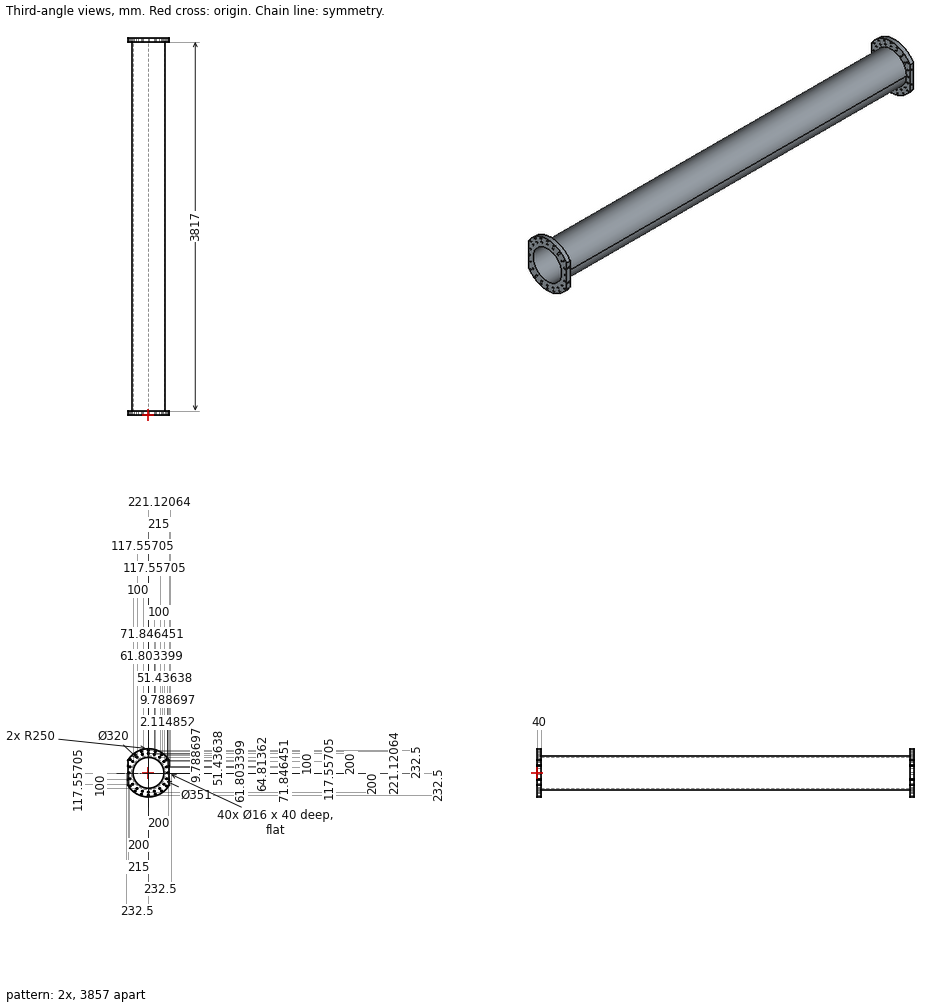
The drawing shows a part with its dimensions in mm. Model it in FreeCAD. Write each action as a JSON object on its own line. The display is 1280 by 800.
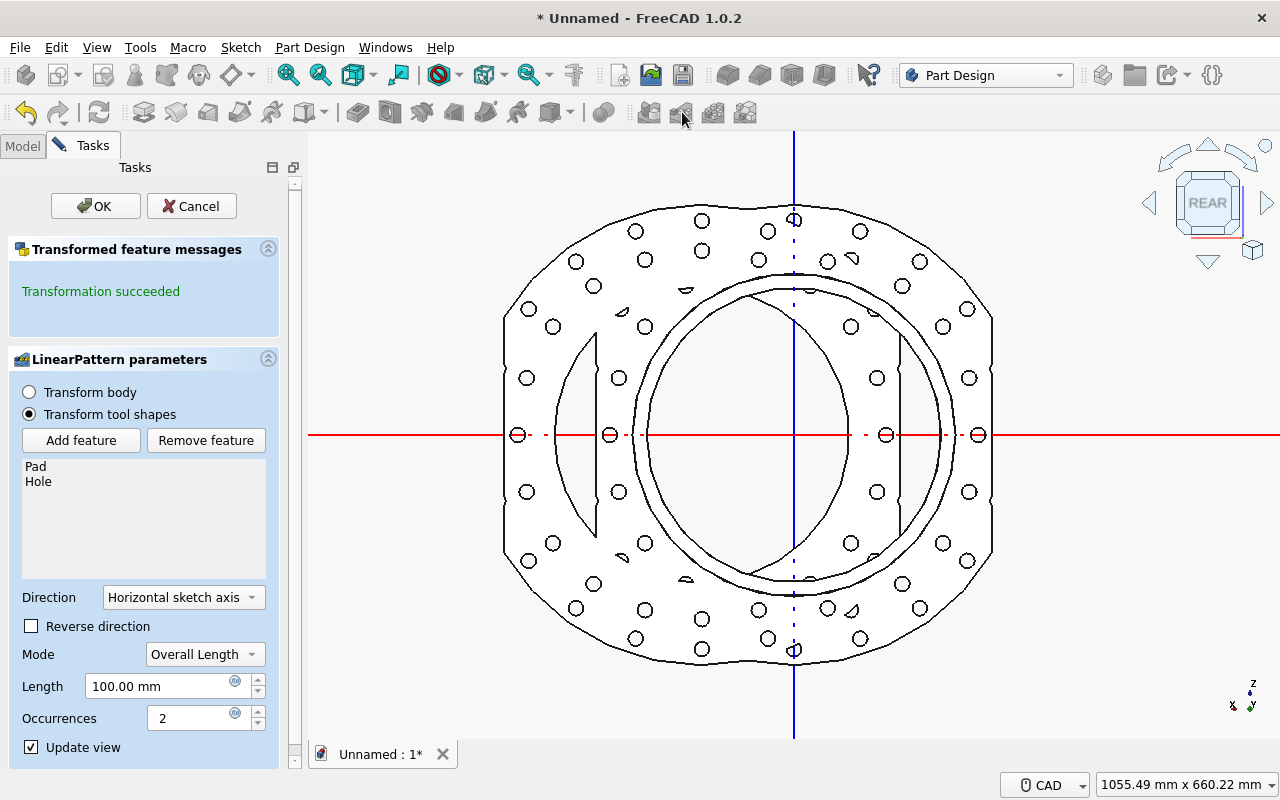
{"action": "left_click", "coordinate": [184, 598]}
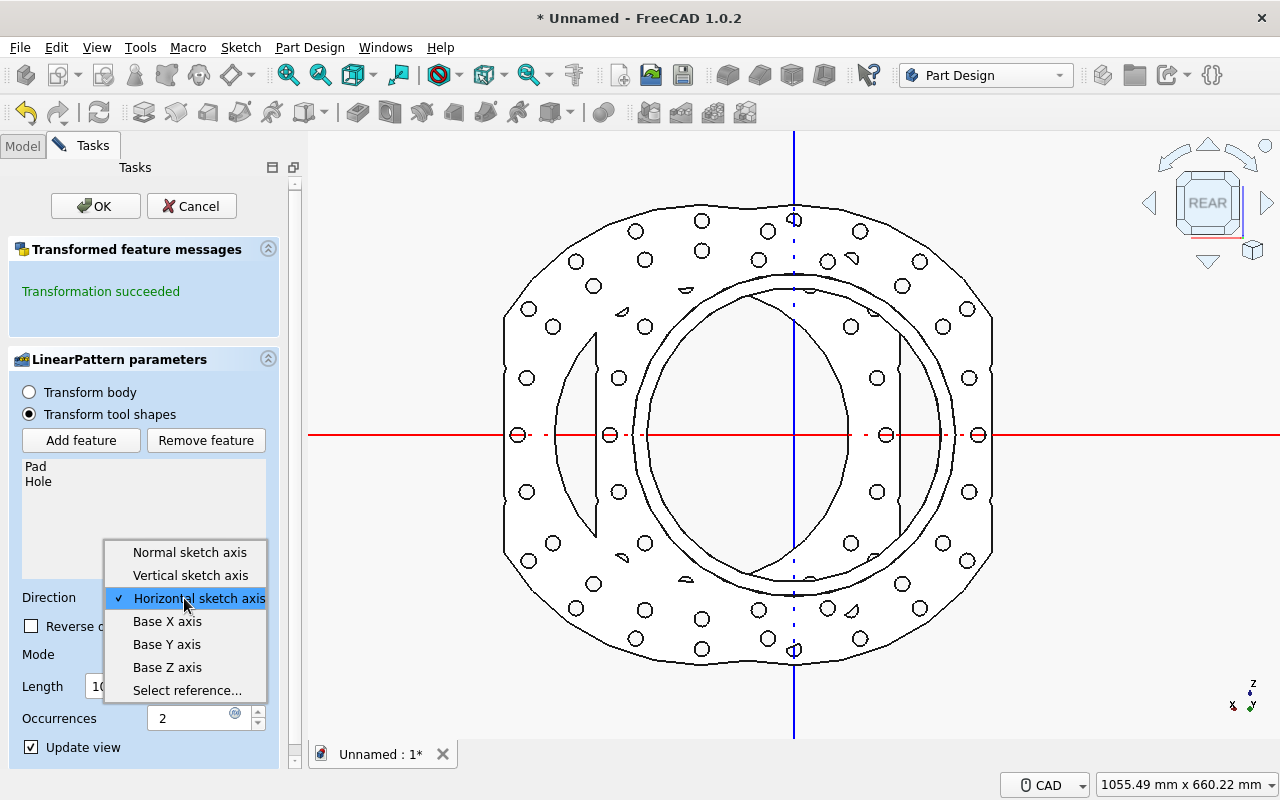
{"action": "left_click", "coordinate": [184, 644]}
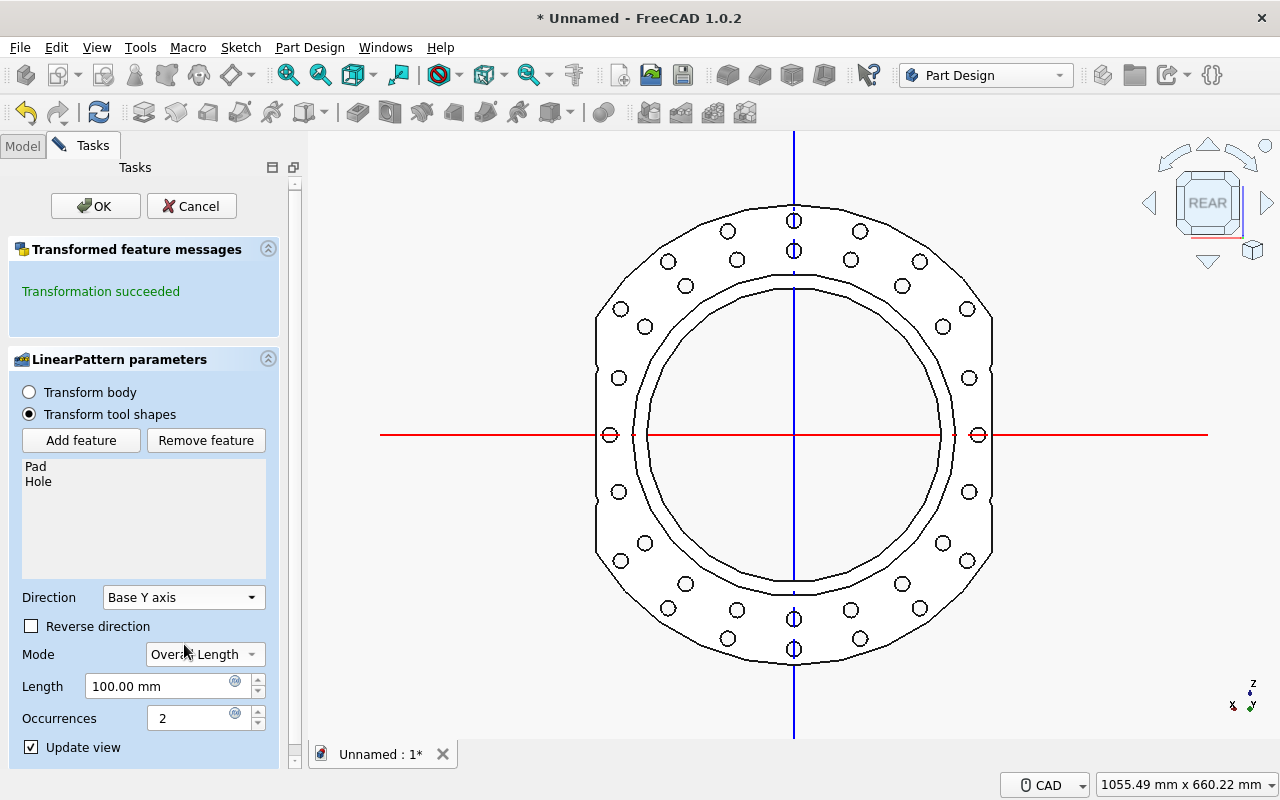
{"action": "left_click", "coordinate": [206, 654]}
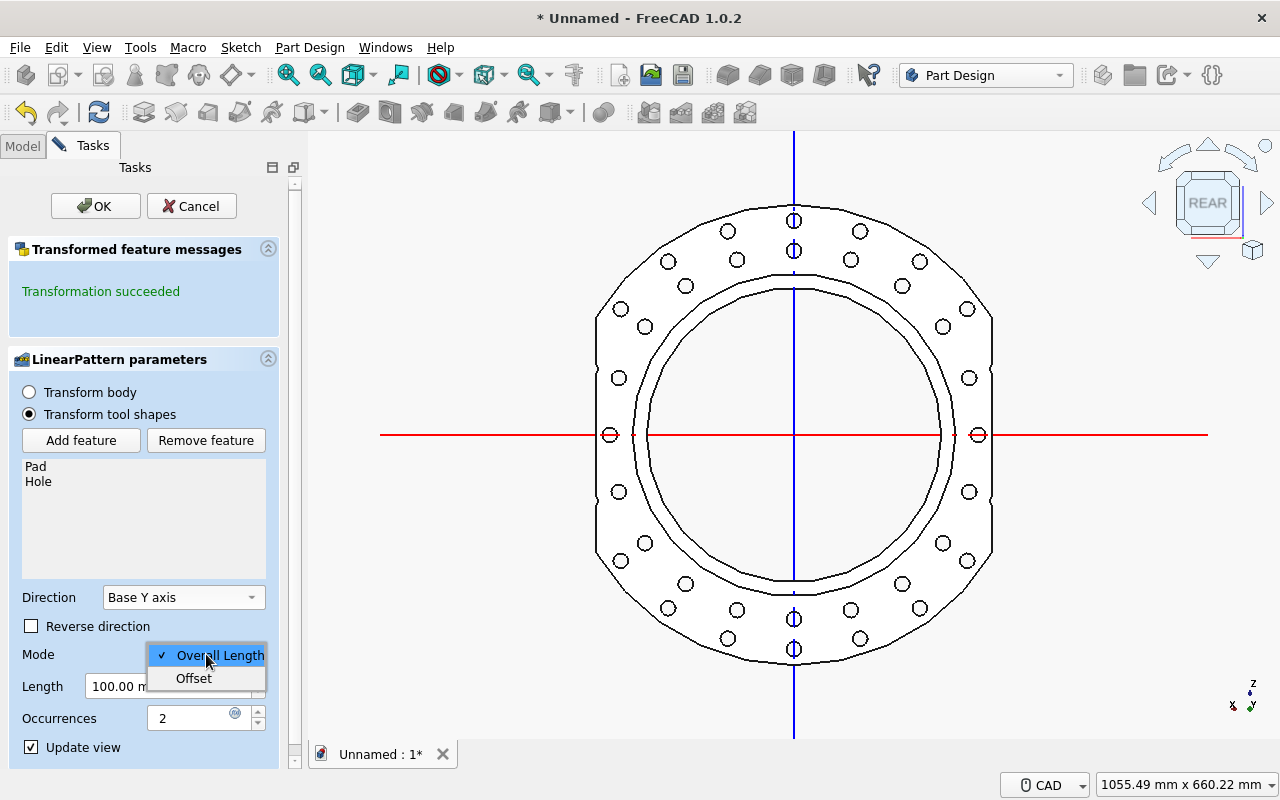
{"action": "left_click", "coordinate": [206, 678]}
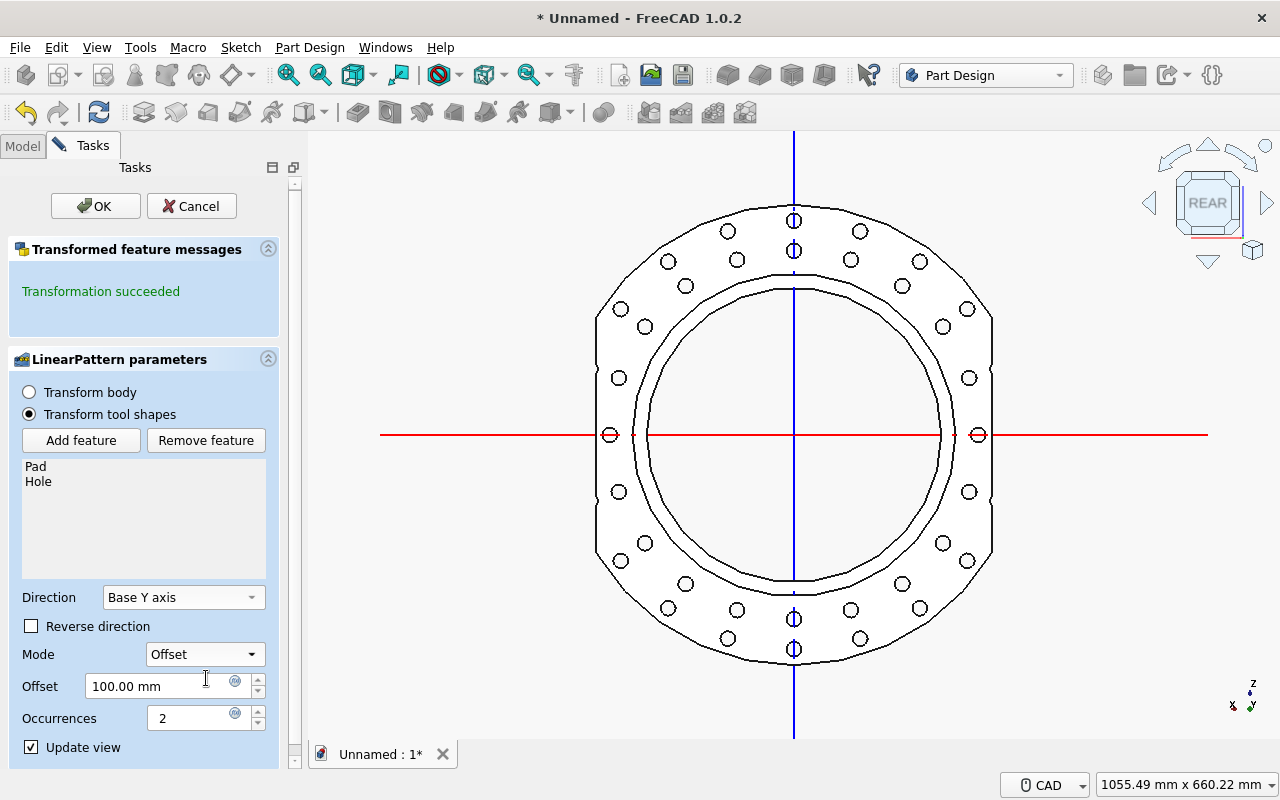
{"action": "triple_click", "coordinate": [168, 686]}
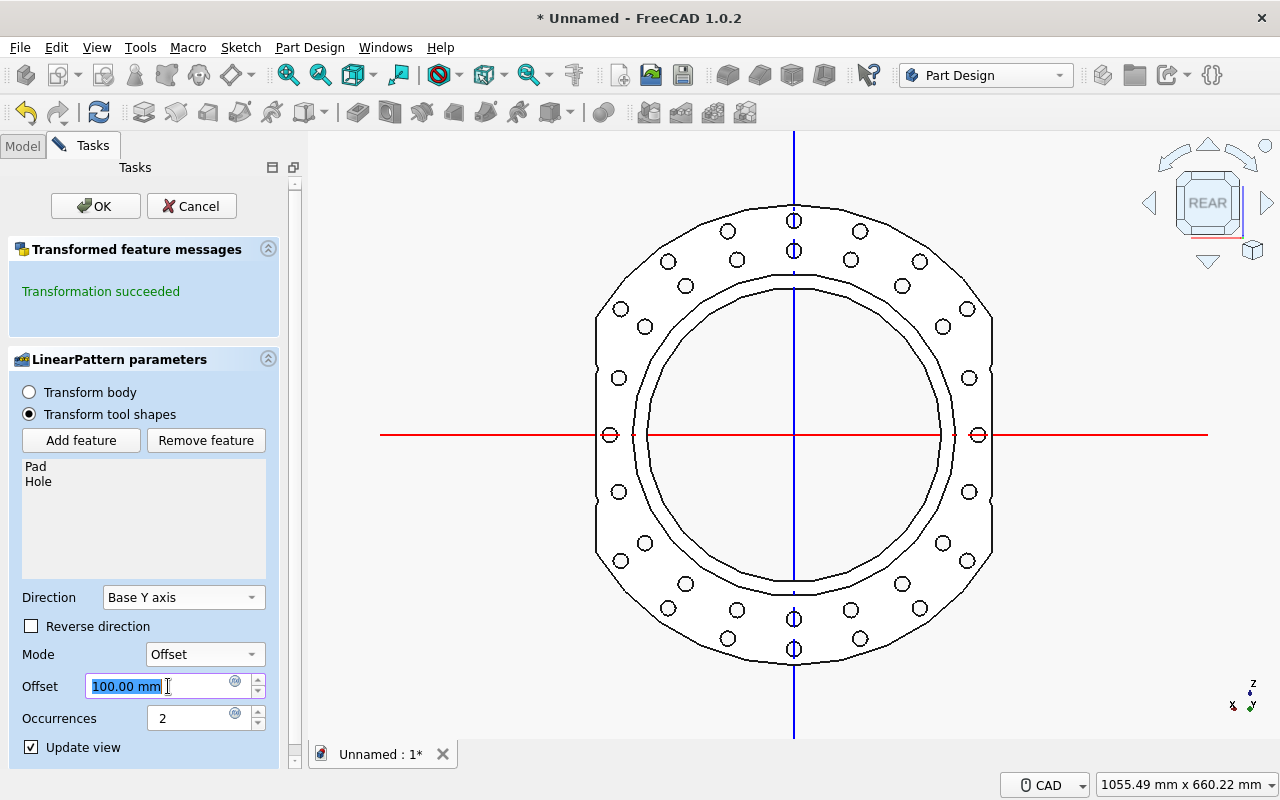
{"action": "type", "text": "3857"}
{"action": "key", "text": "Tab"}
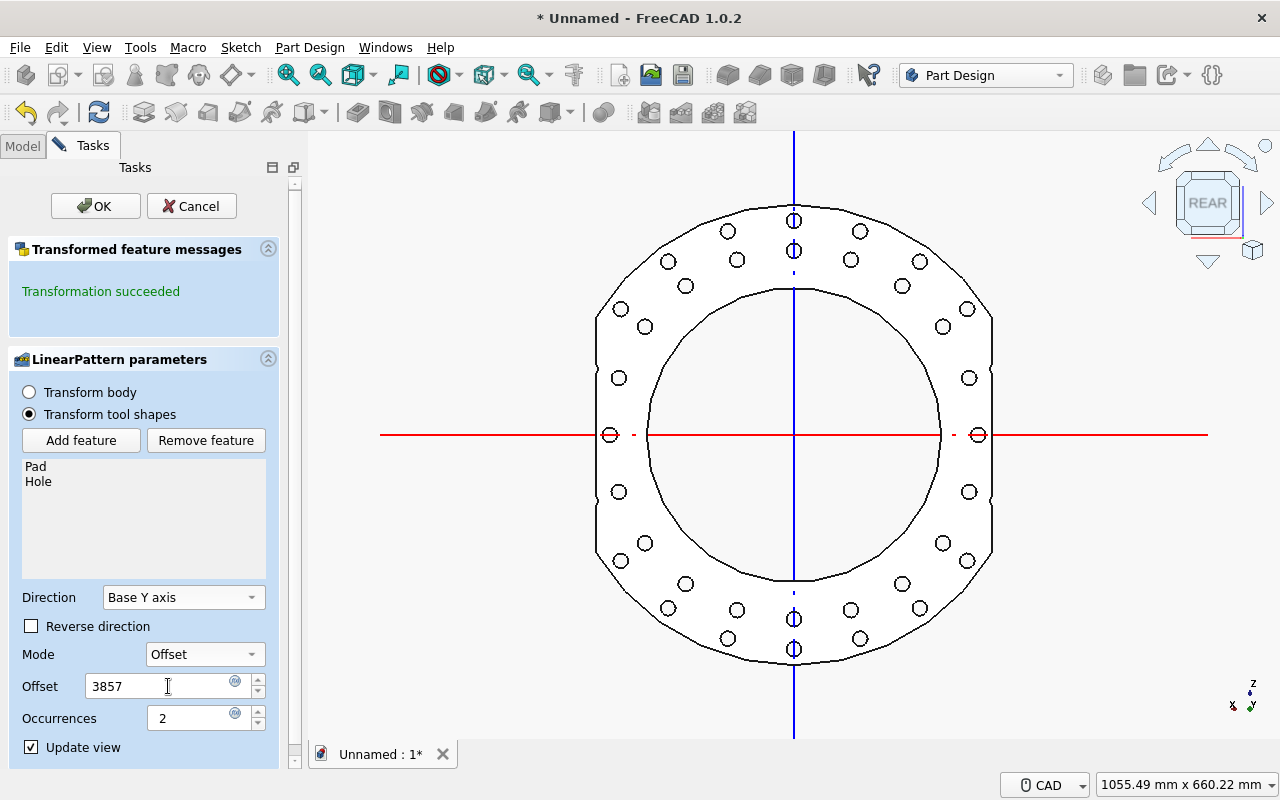
{"action": "triple_click", "coordinate": [198, 718]}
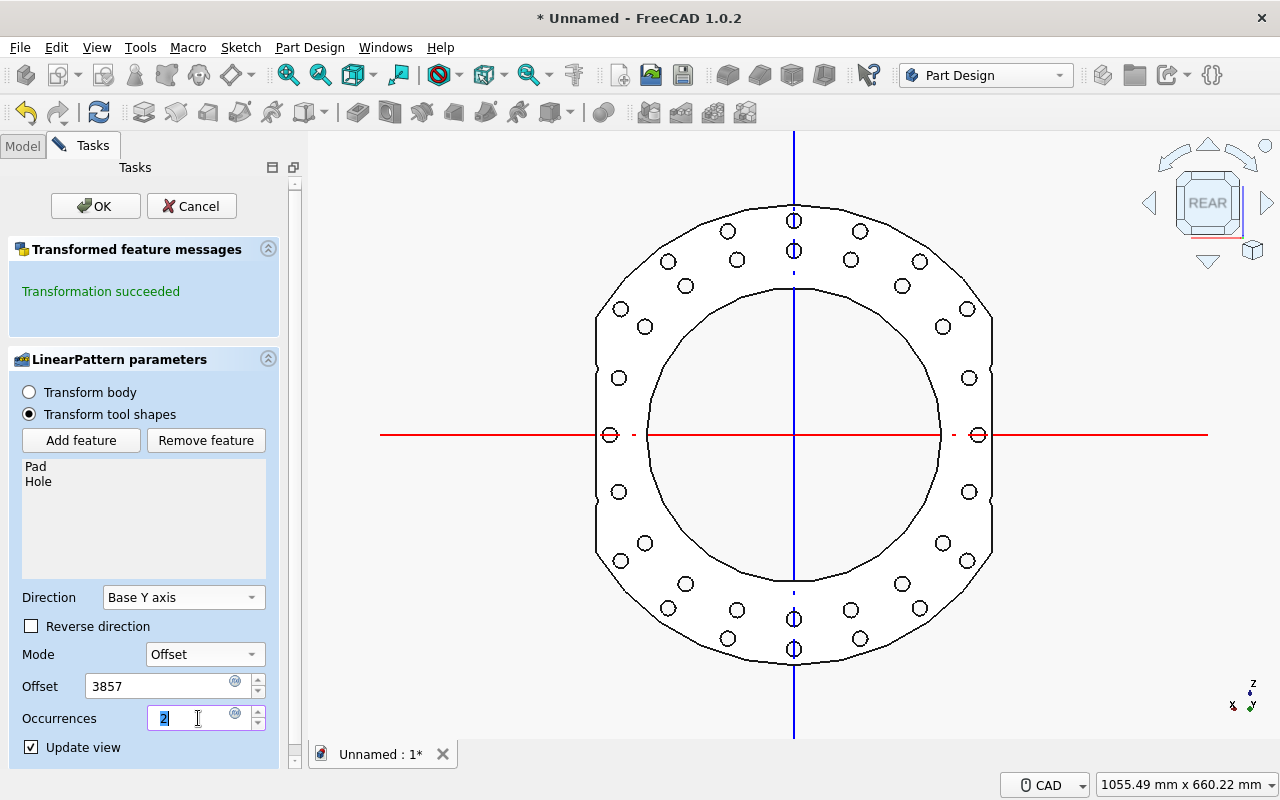
{"action": "type", "text": "2"}
{"action": "key", "text": "Tab"}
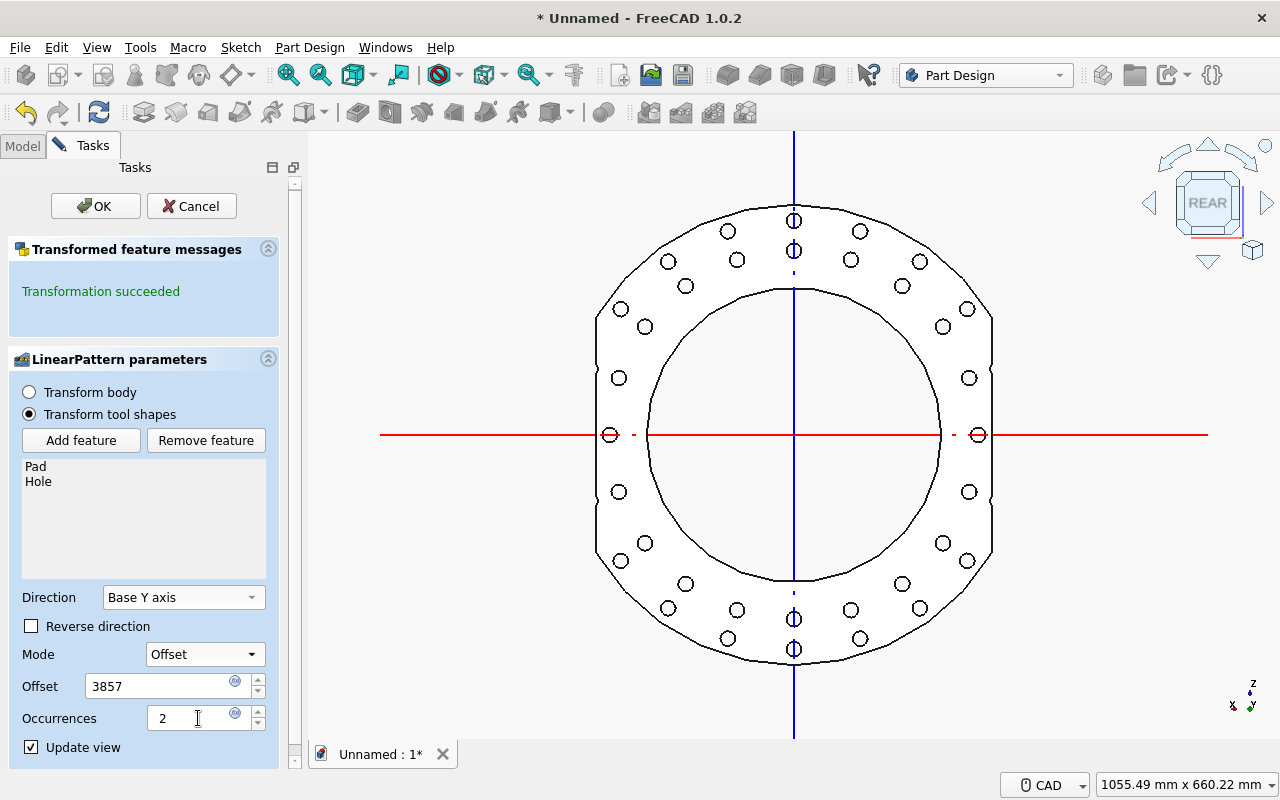
{"action": "left_click", "coordinate": [96, 206]}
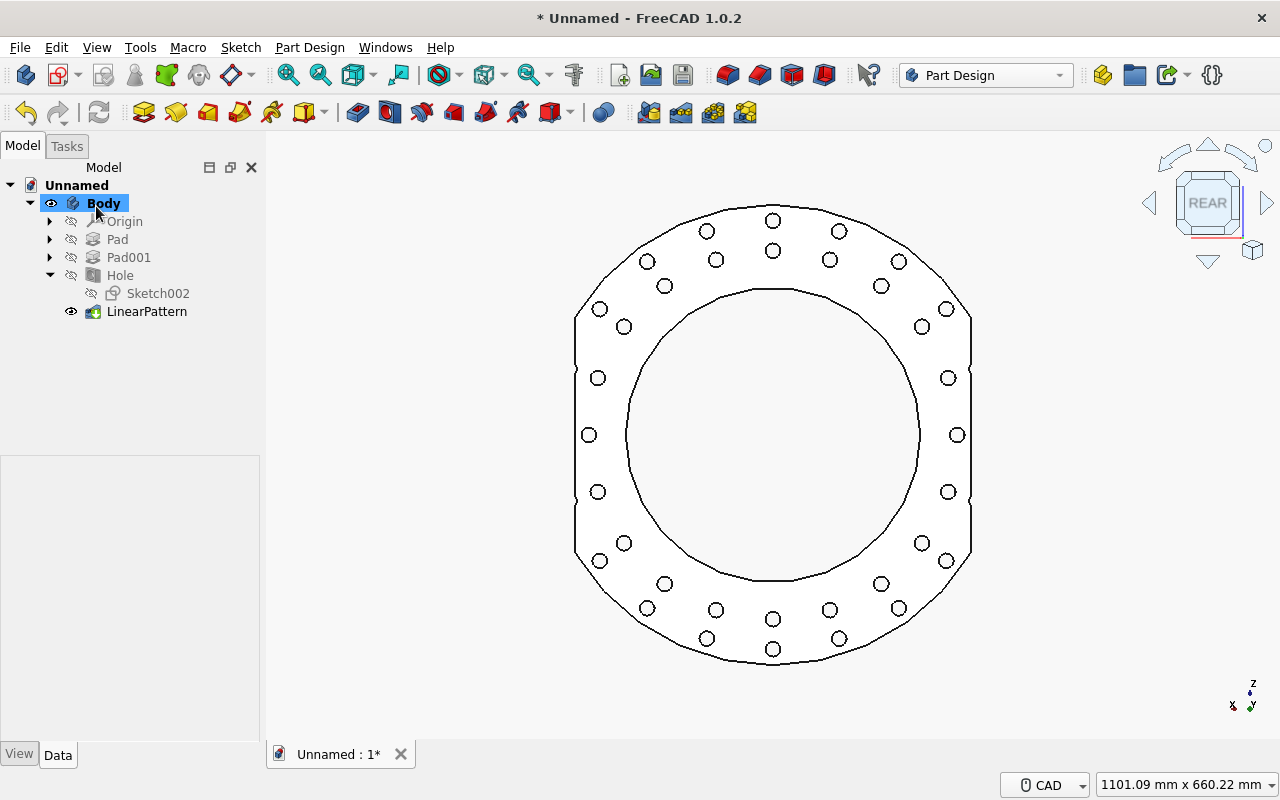
{"action": "key", "text": "0"}